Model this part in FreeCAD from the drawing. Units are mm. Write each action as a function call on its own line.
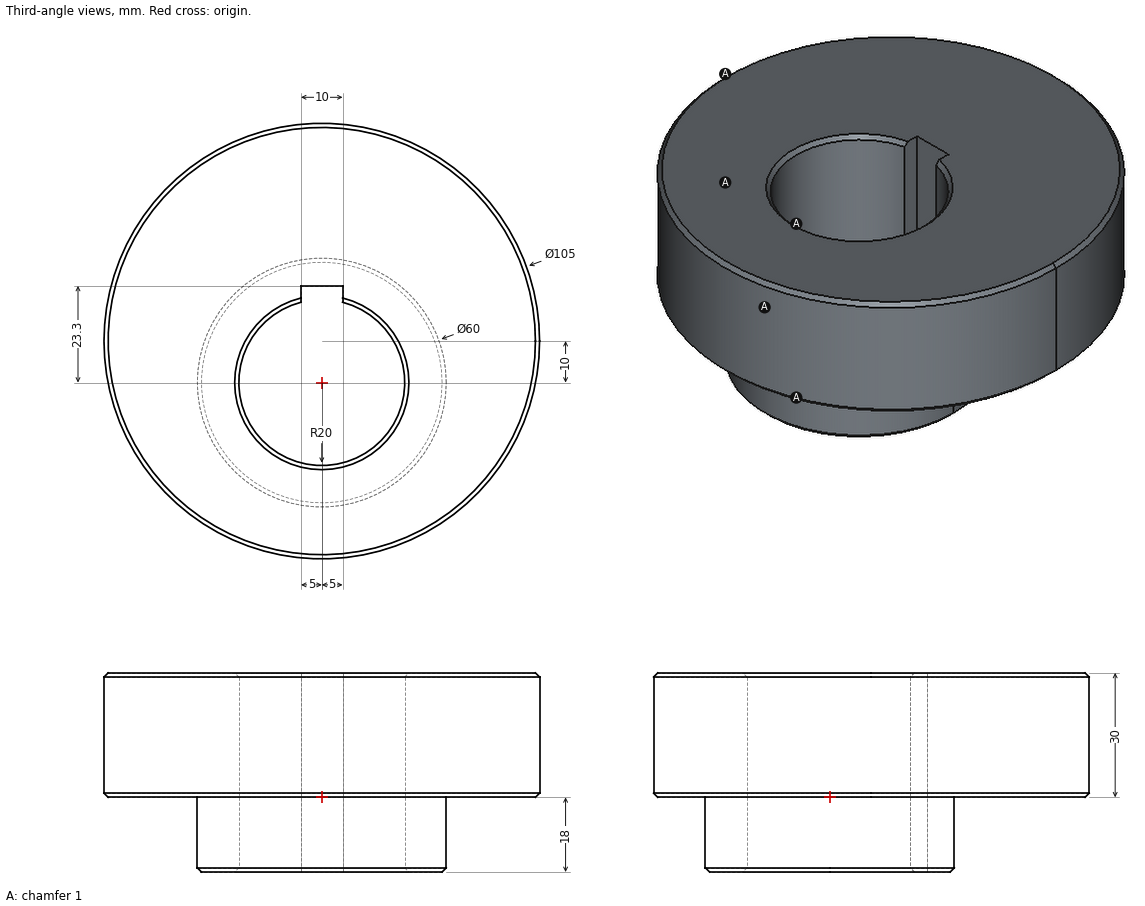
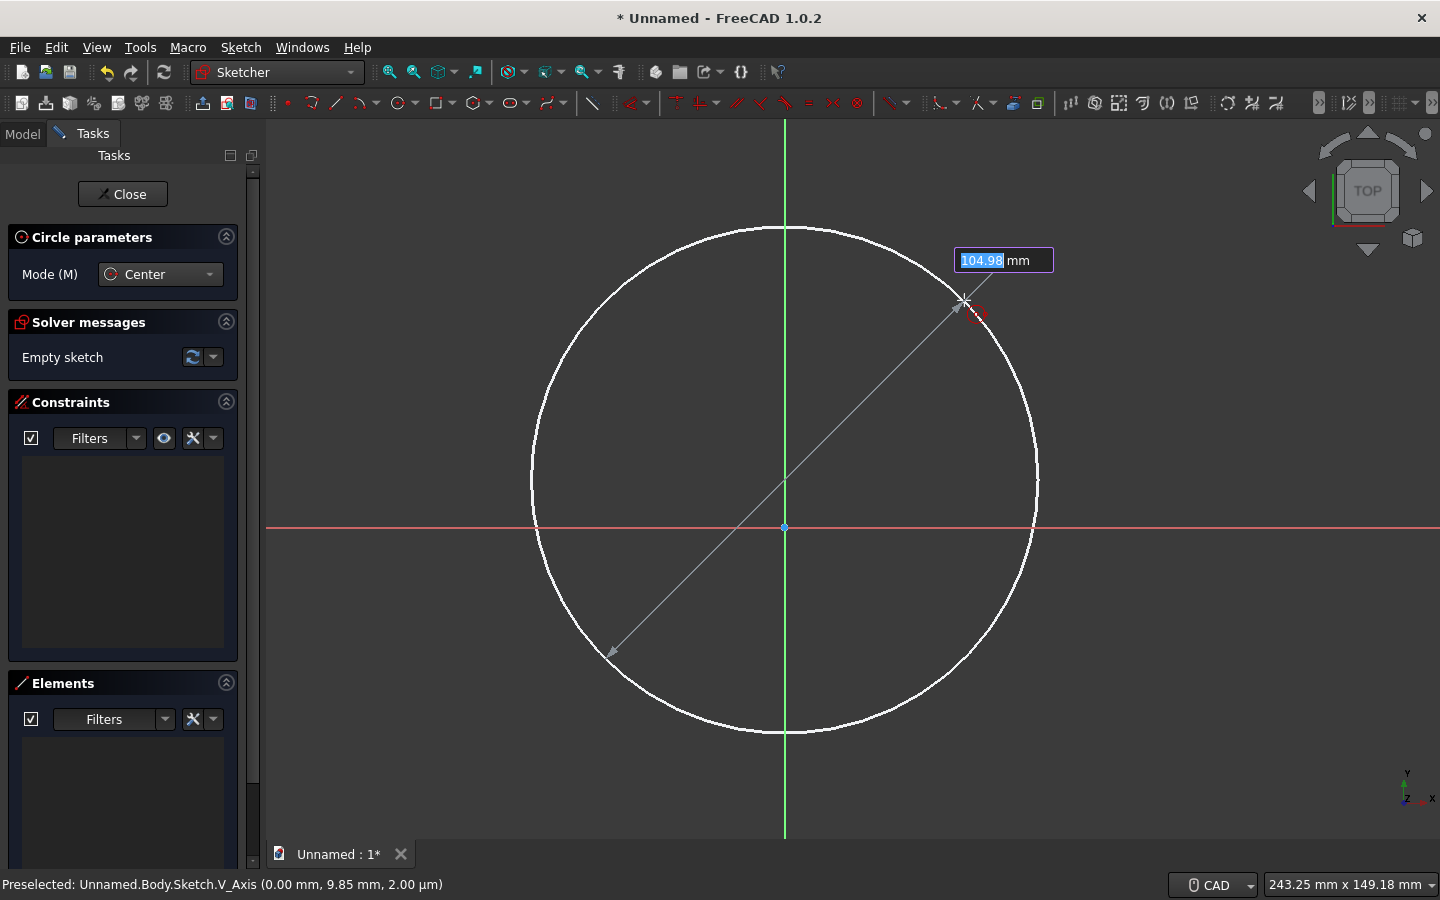
text(105)
key(Return)
key(Escape)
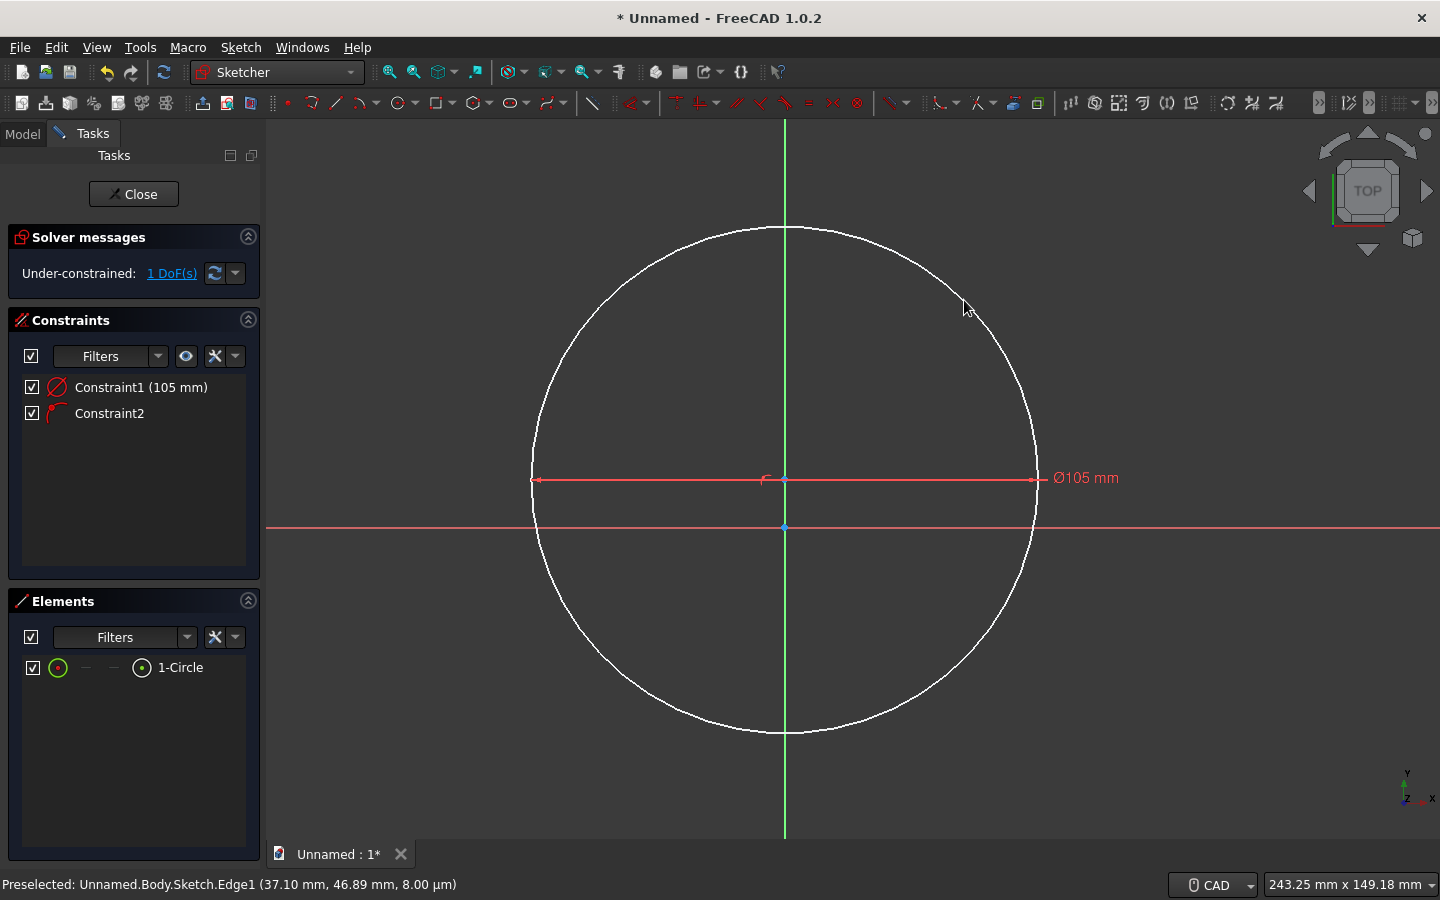
click(630, 104)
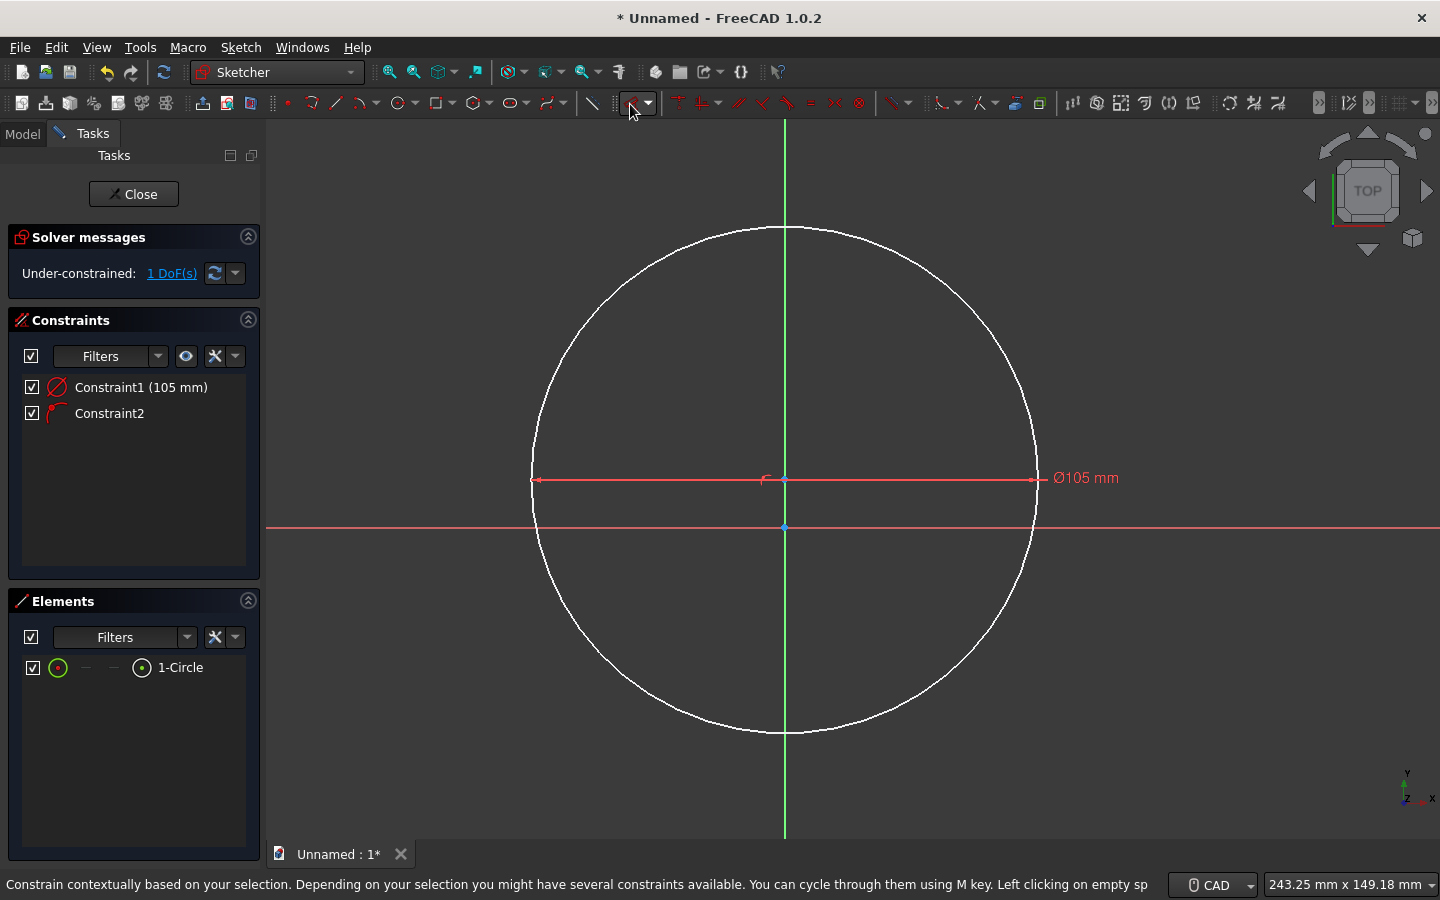
click(785, 480)
click(819, 504)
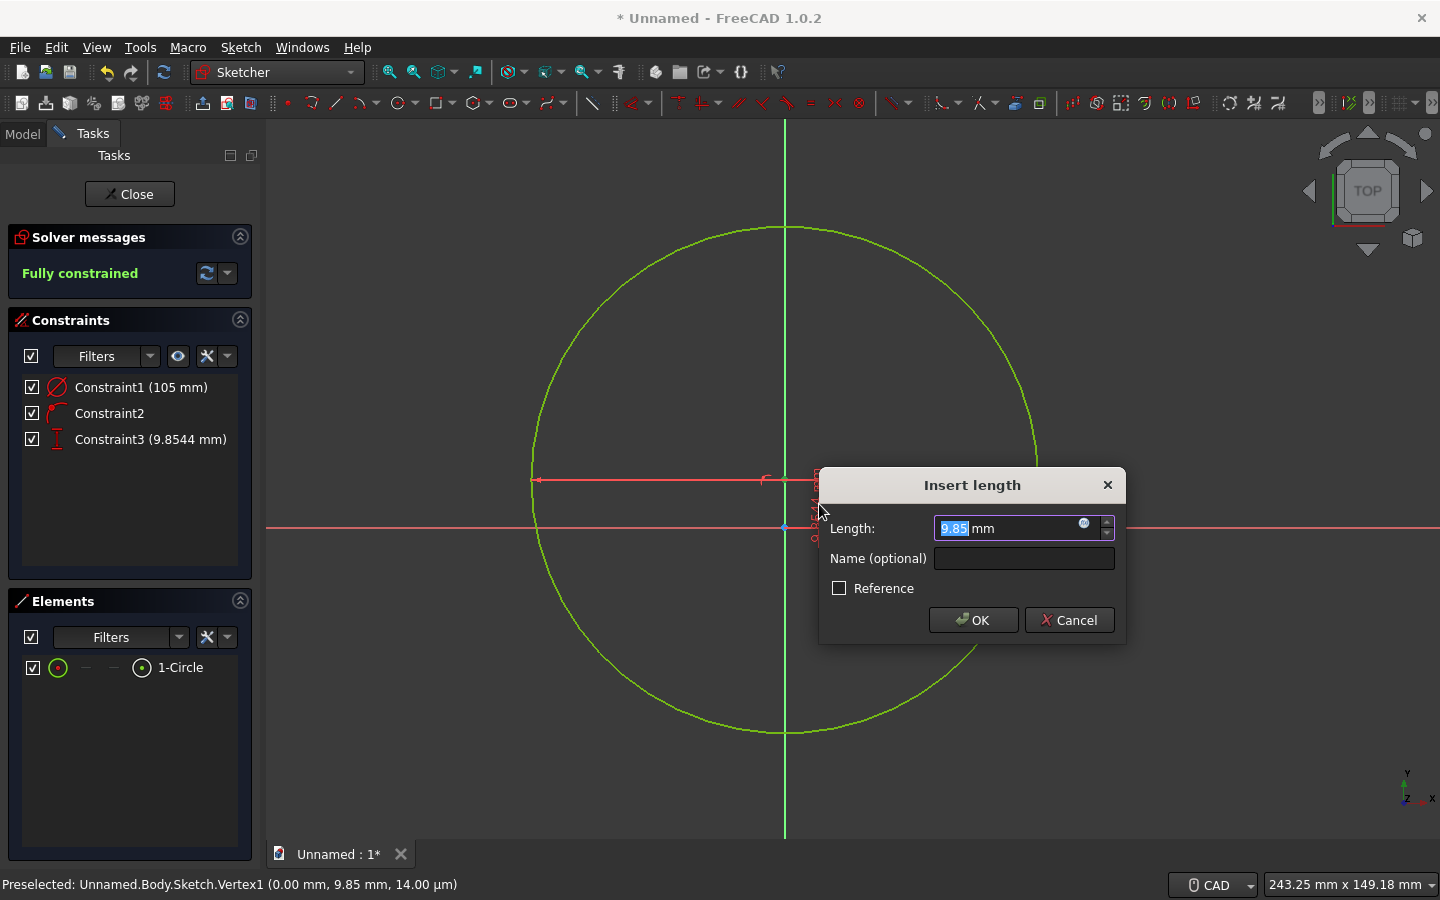
text(10)
key(Return)
key(Escape)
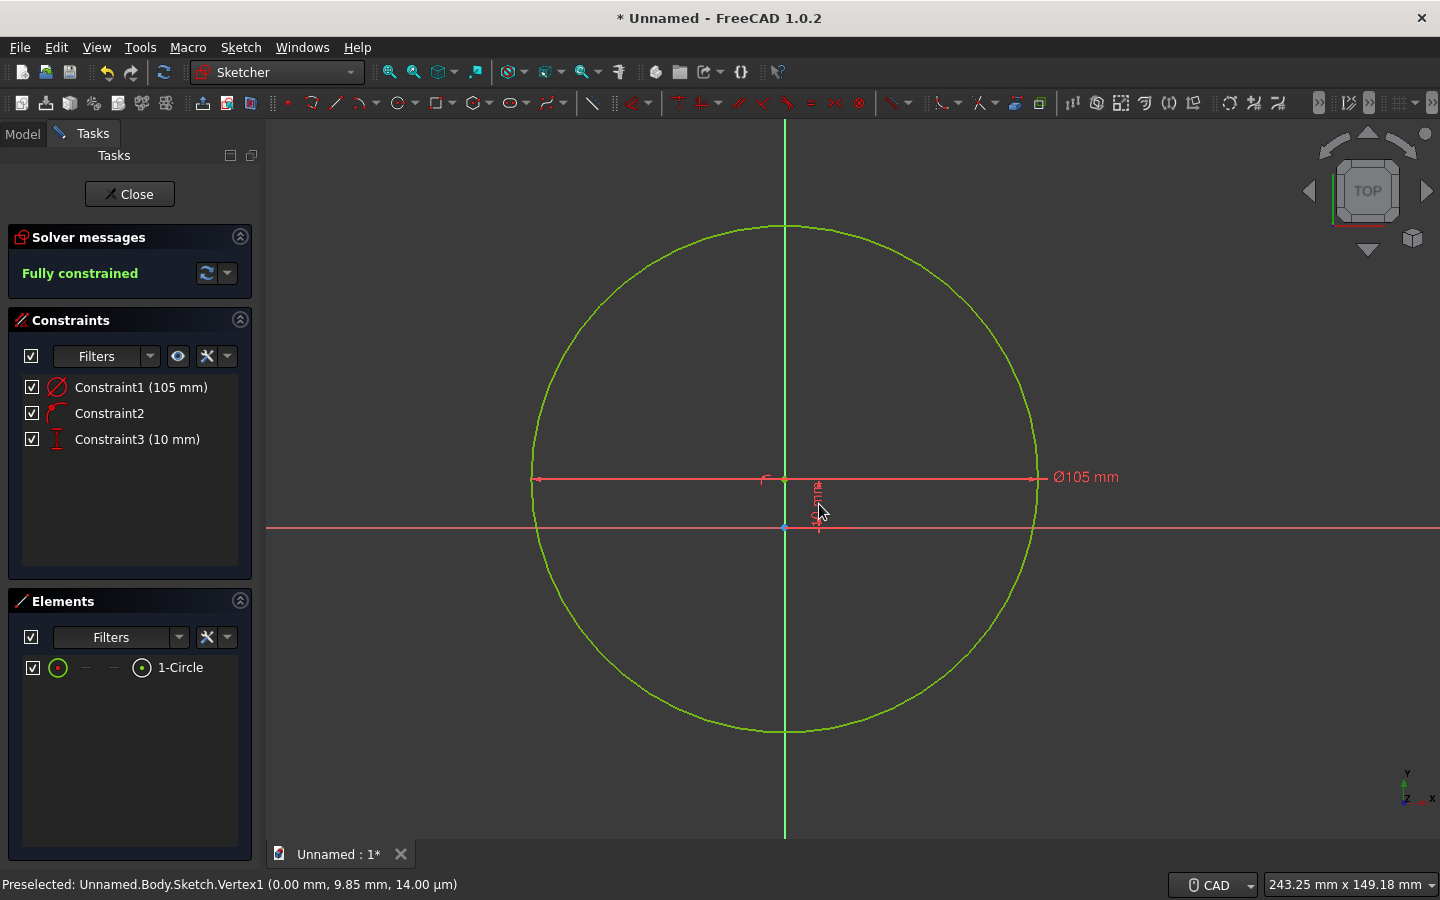
click(130, 194)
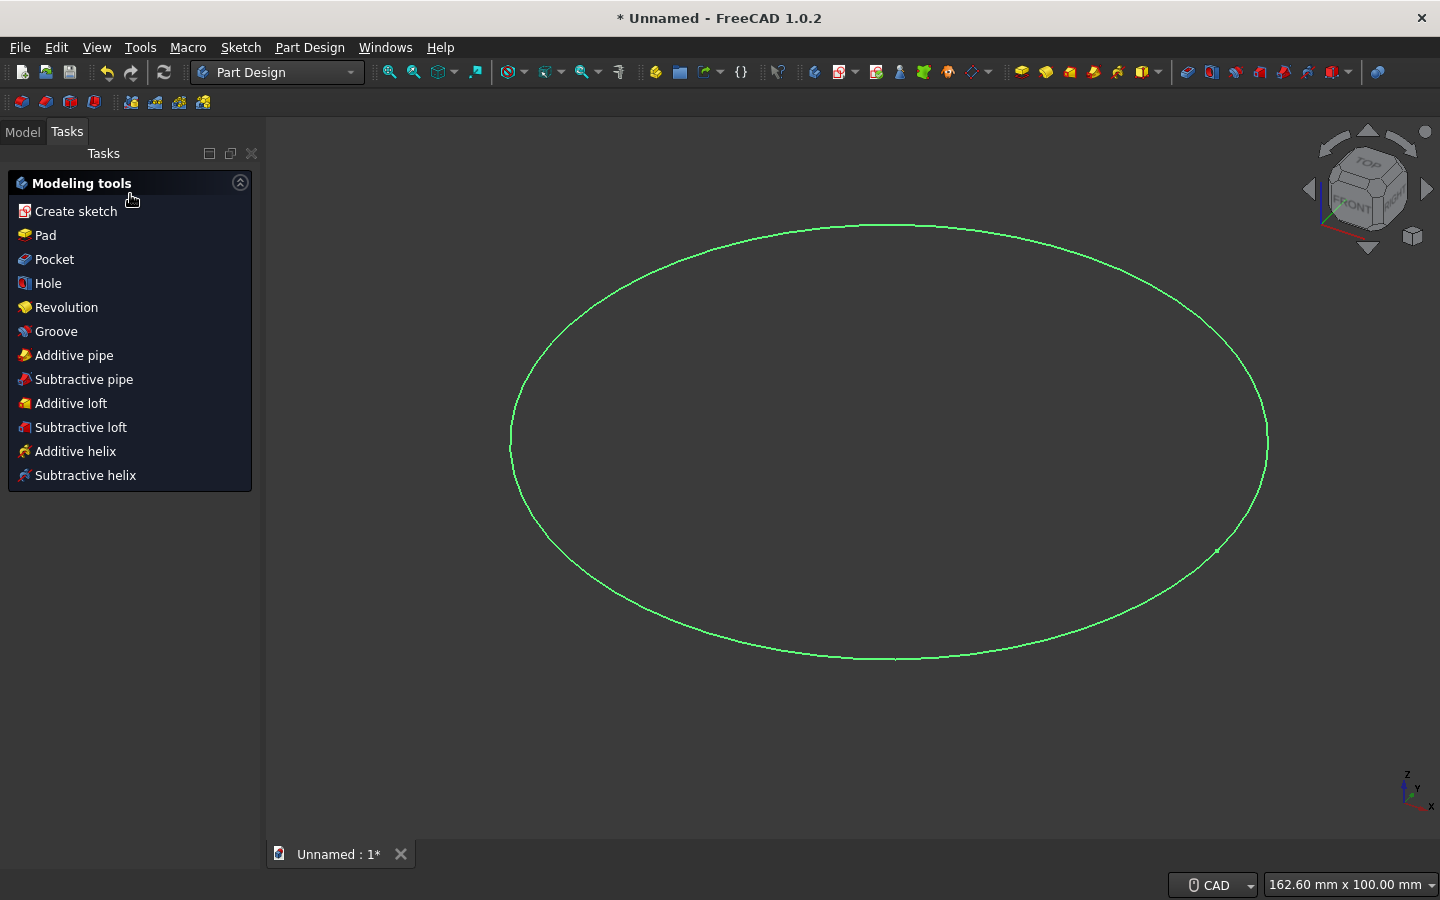
click(1022, 72)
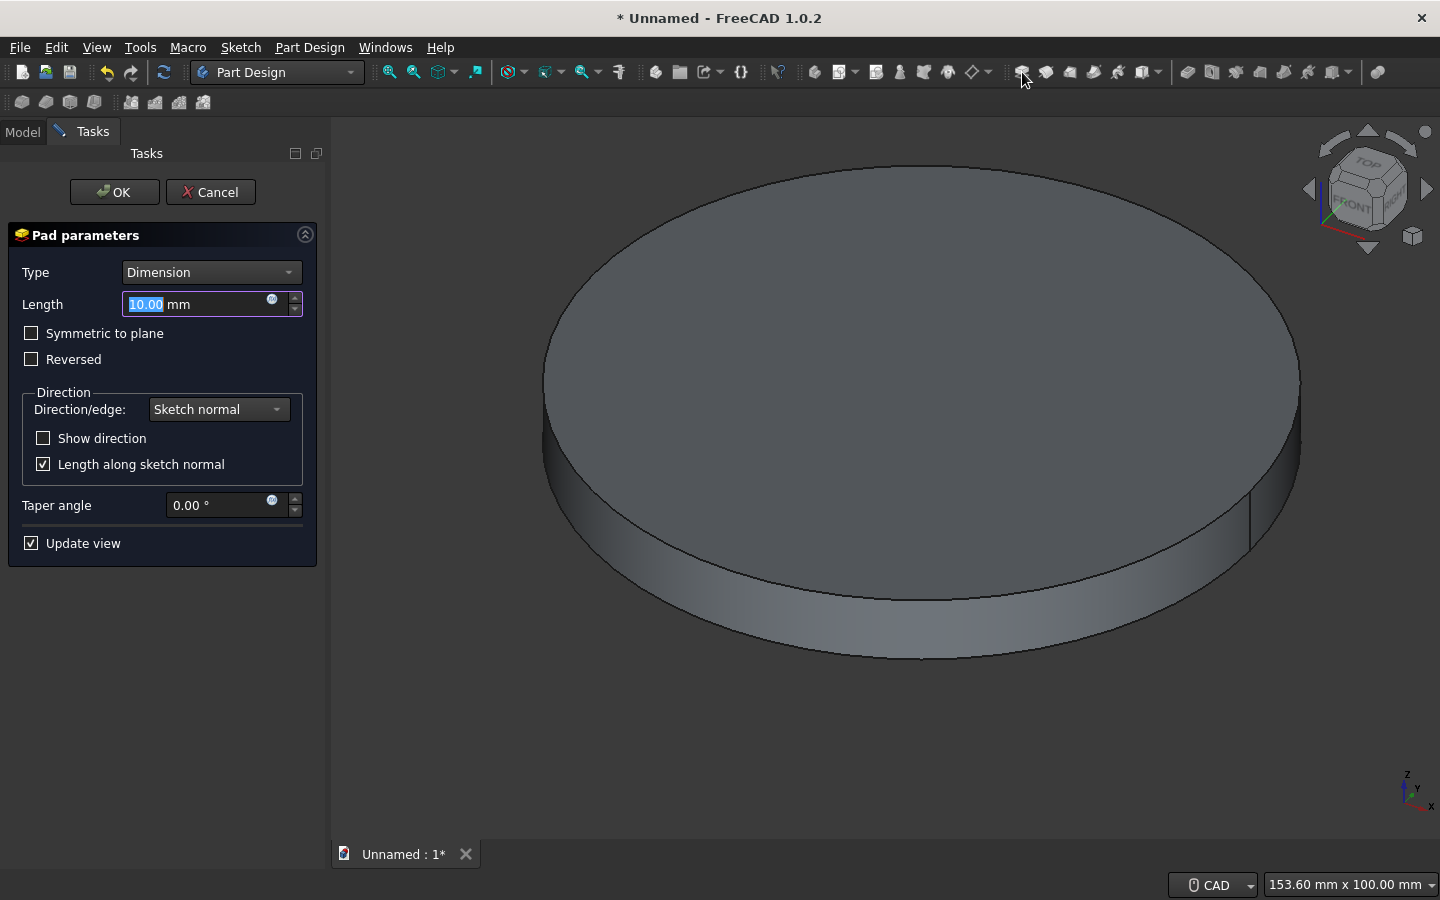
text(30)
key(Tab)